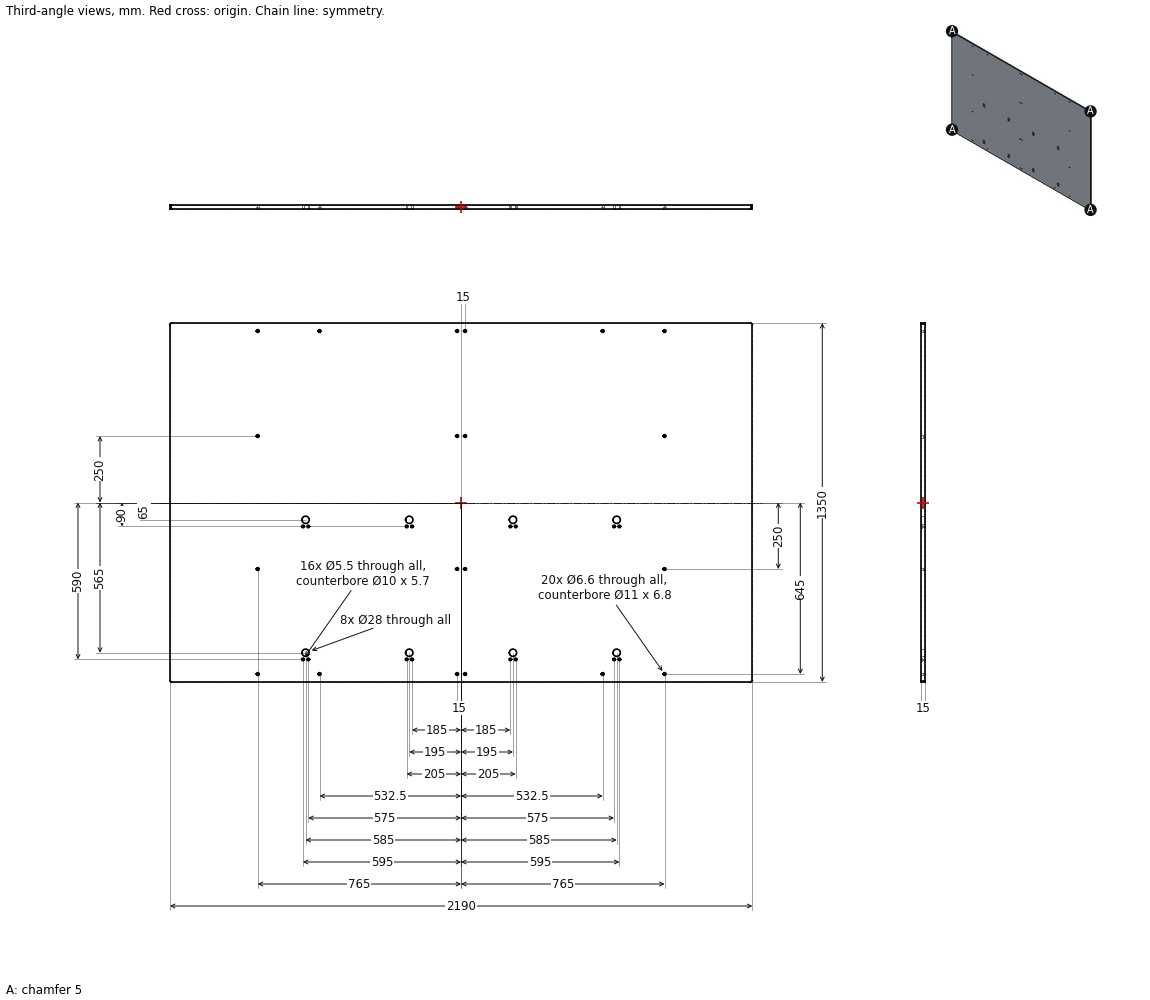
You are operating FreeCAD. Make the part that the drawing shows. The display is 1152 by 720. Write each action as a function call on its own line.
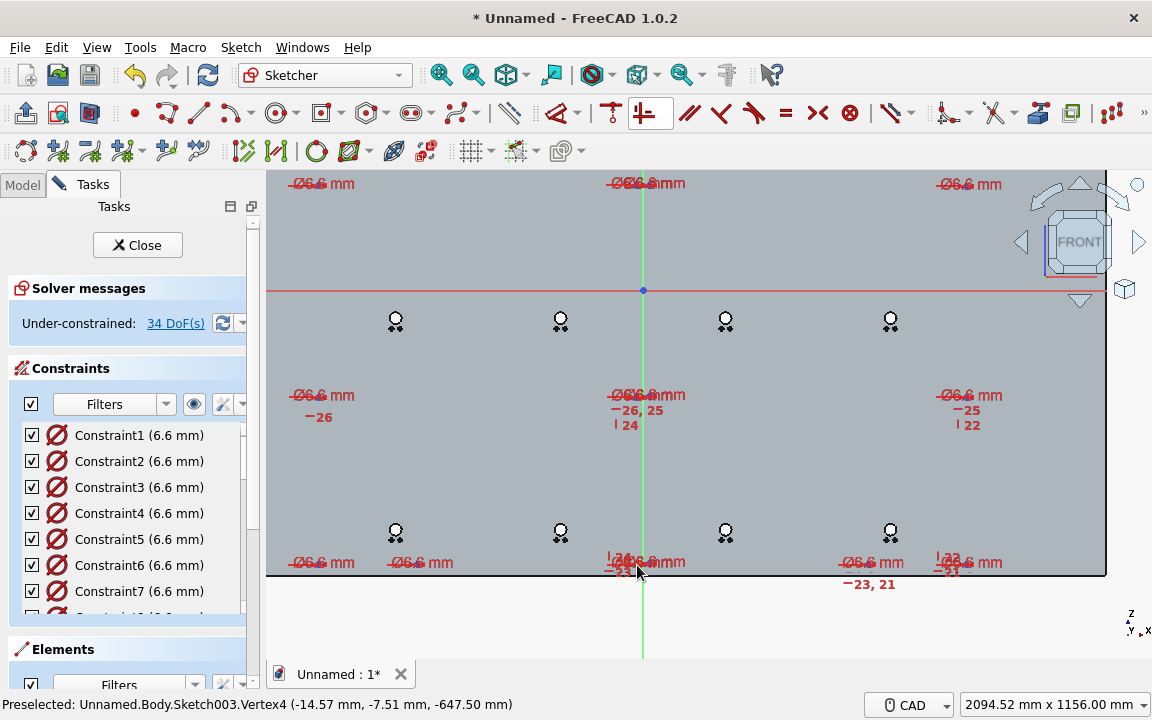
click(417, 565)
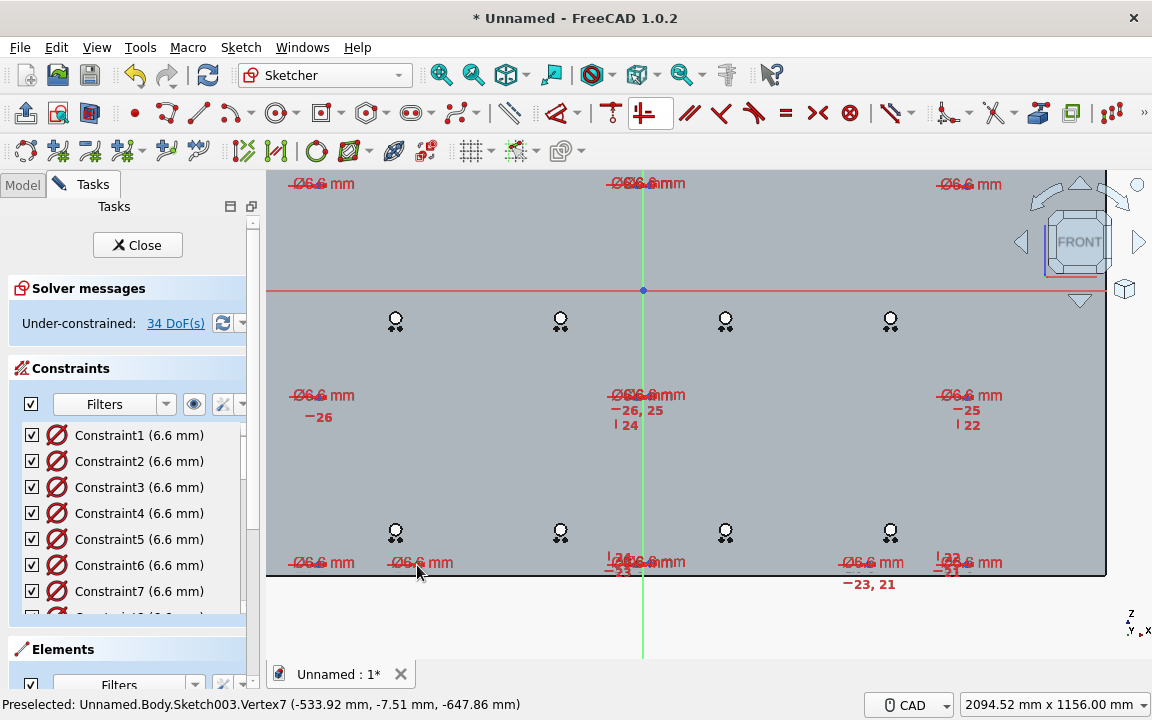
key(h)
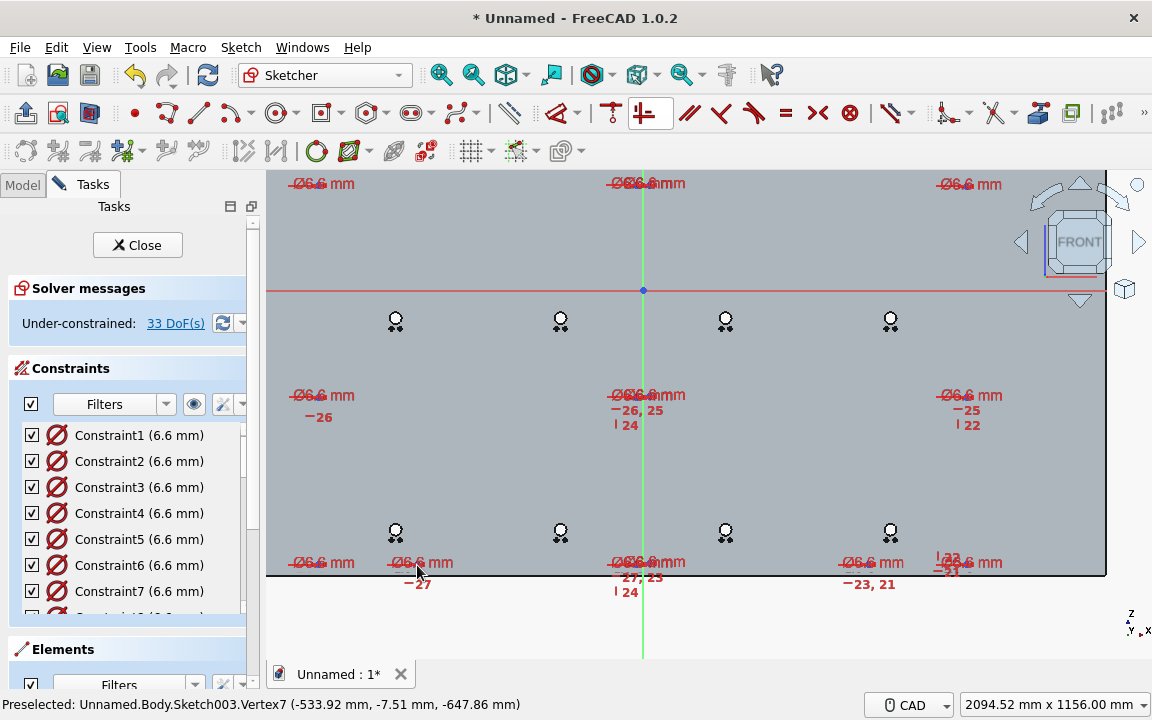
click(319, 397)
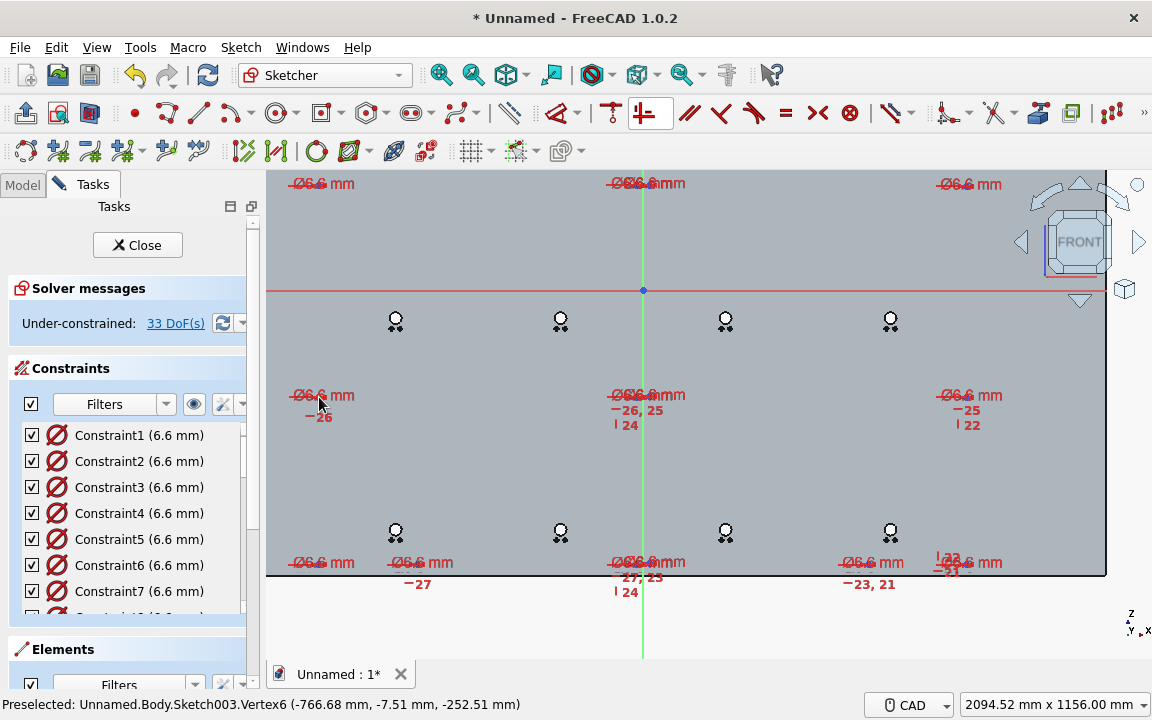
click(319, 565)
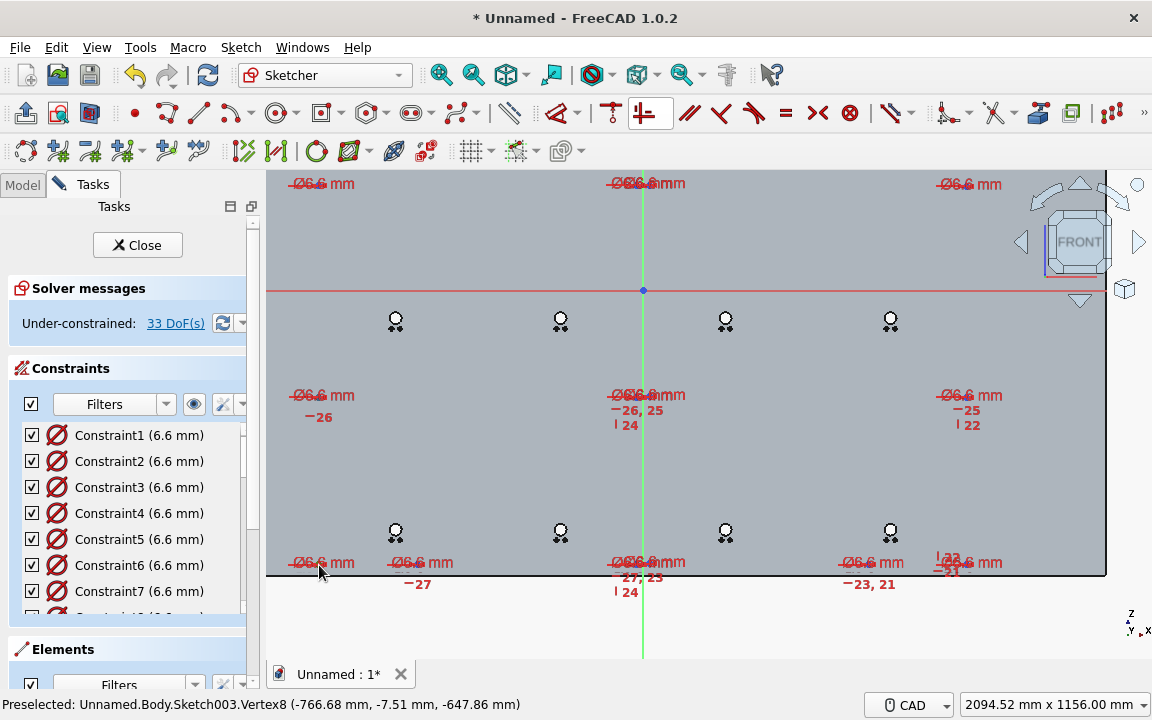
key(v)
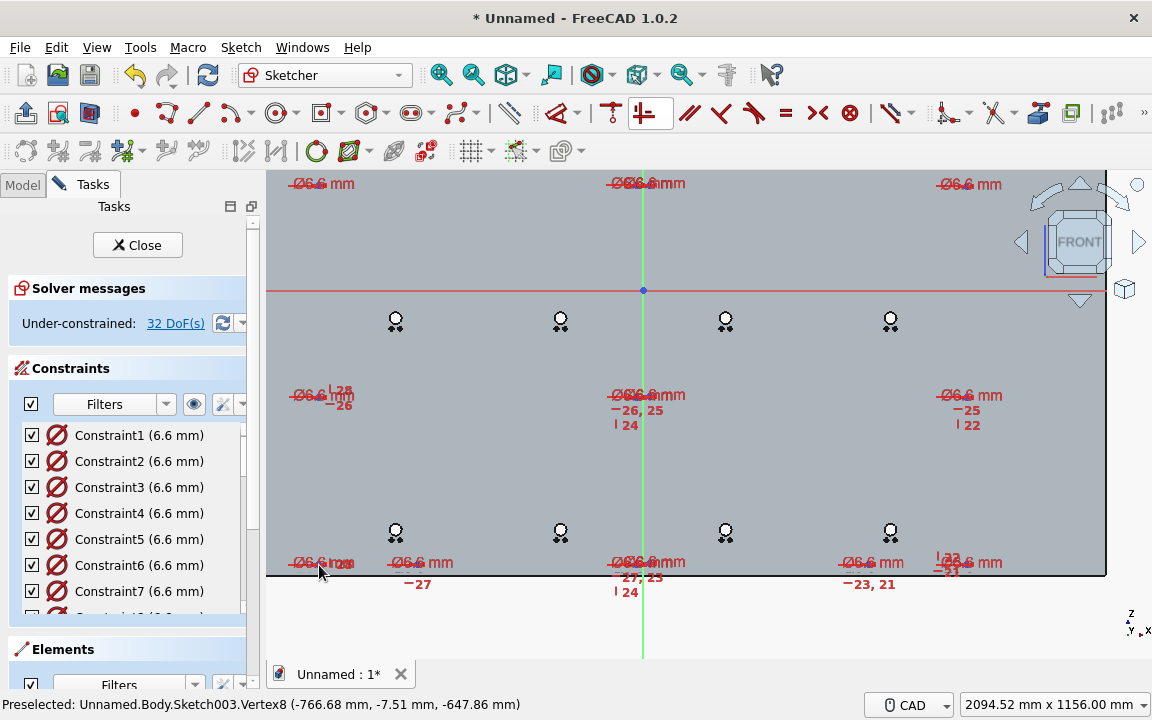
click(417, 565)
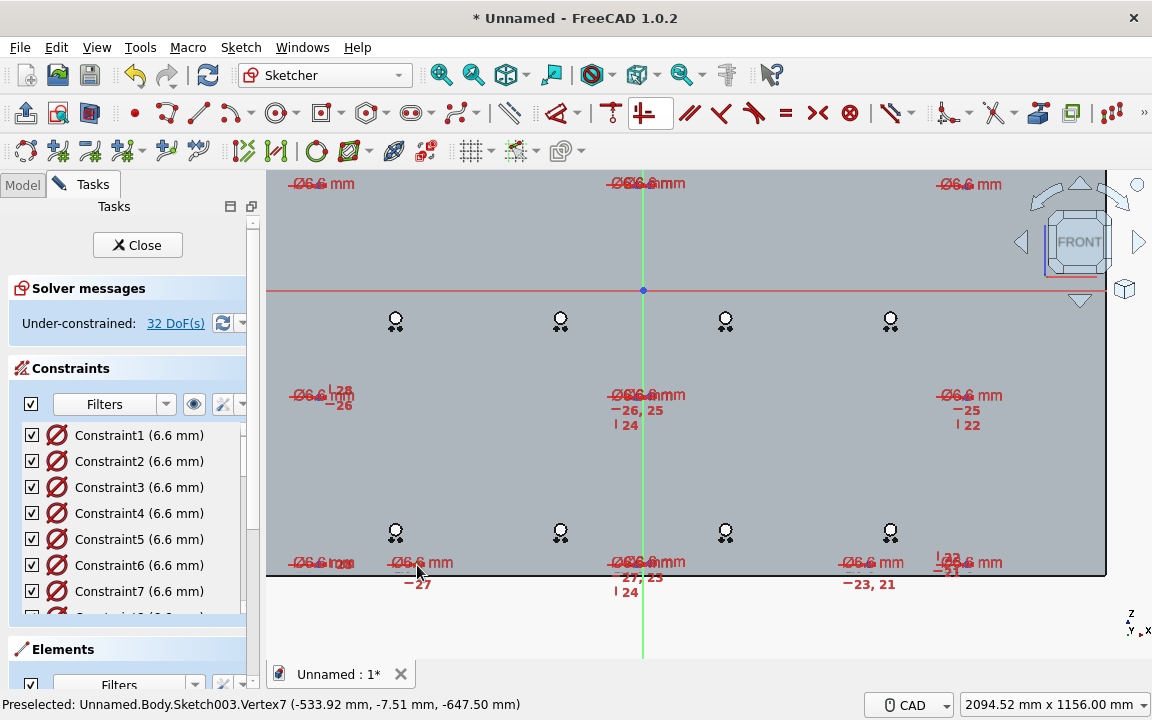
click(319, 565)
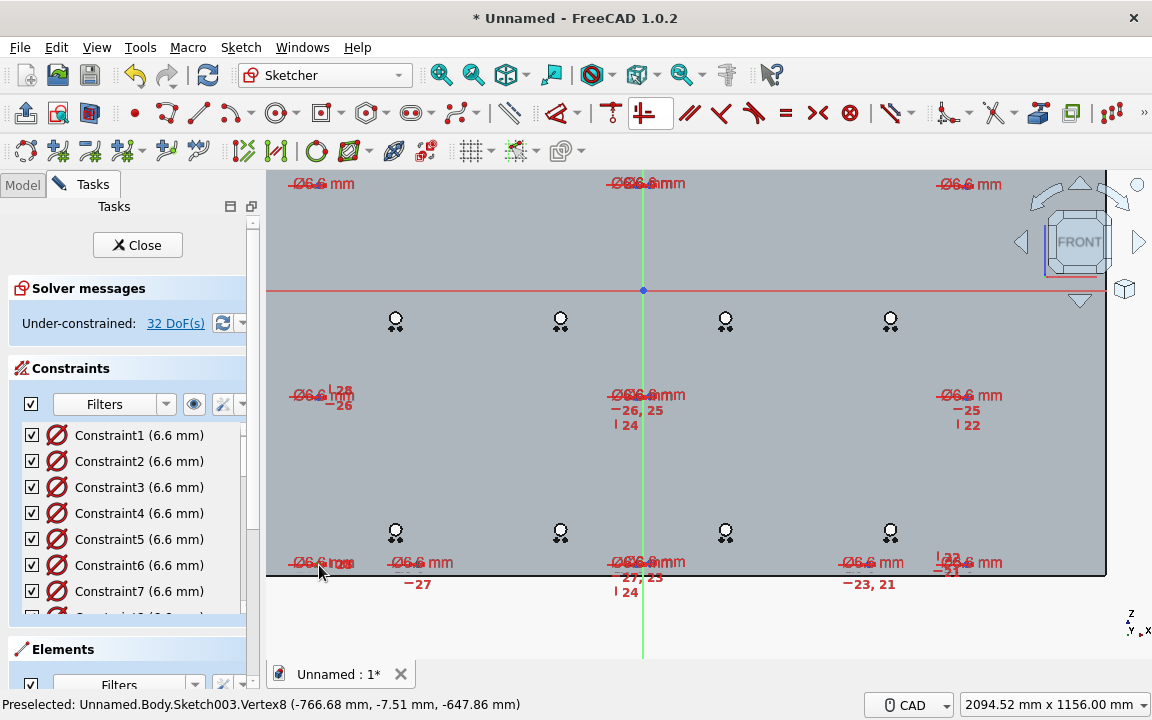
key(h)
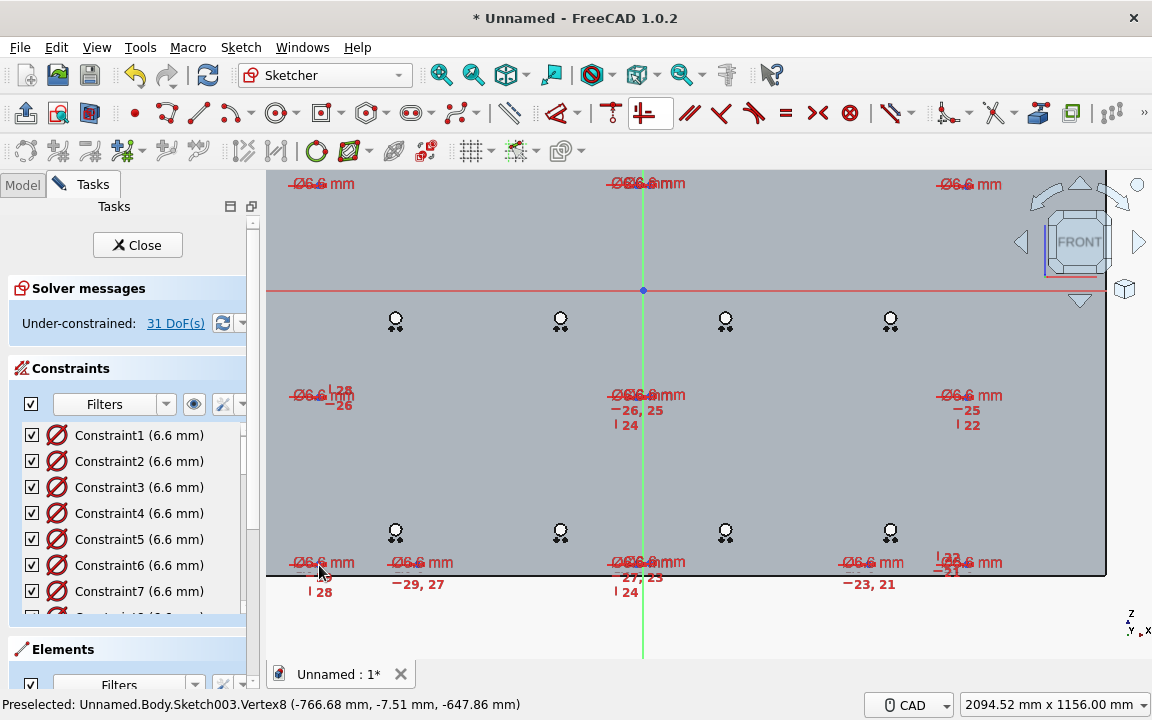
click(319, 397)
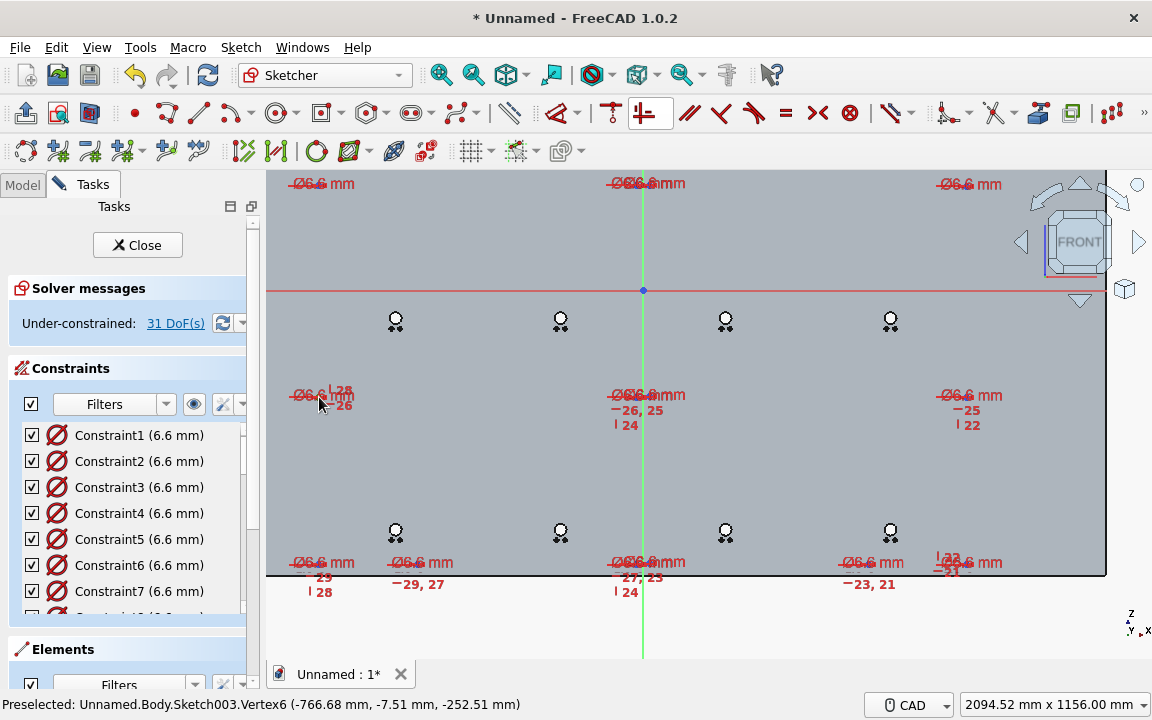
scroll(637, 565, down, 3)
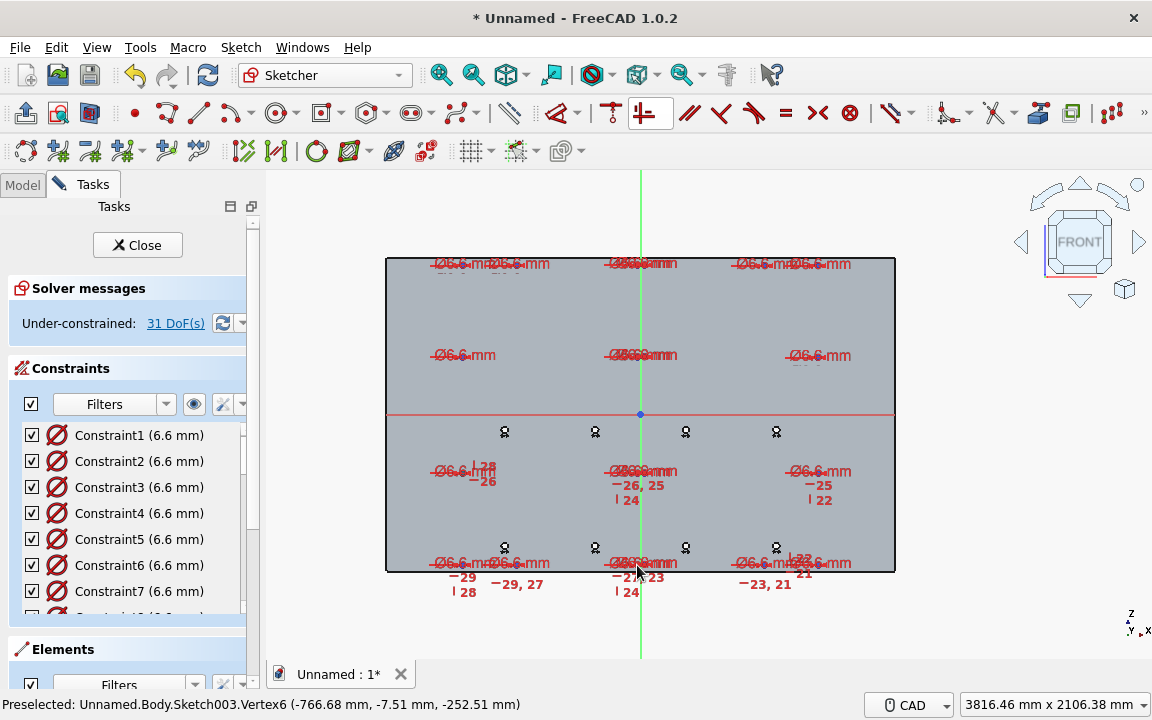
click(463, 266)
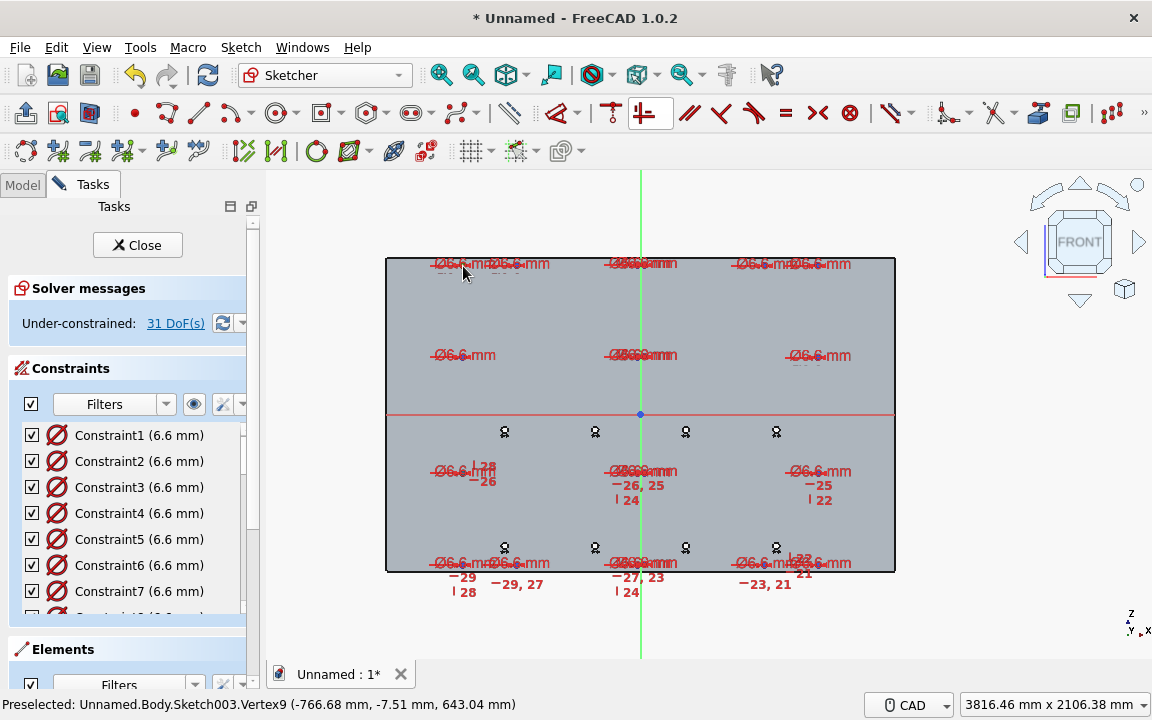
key(v)